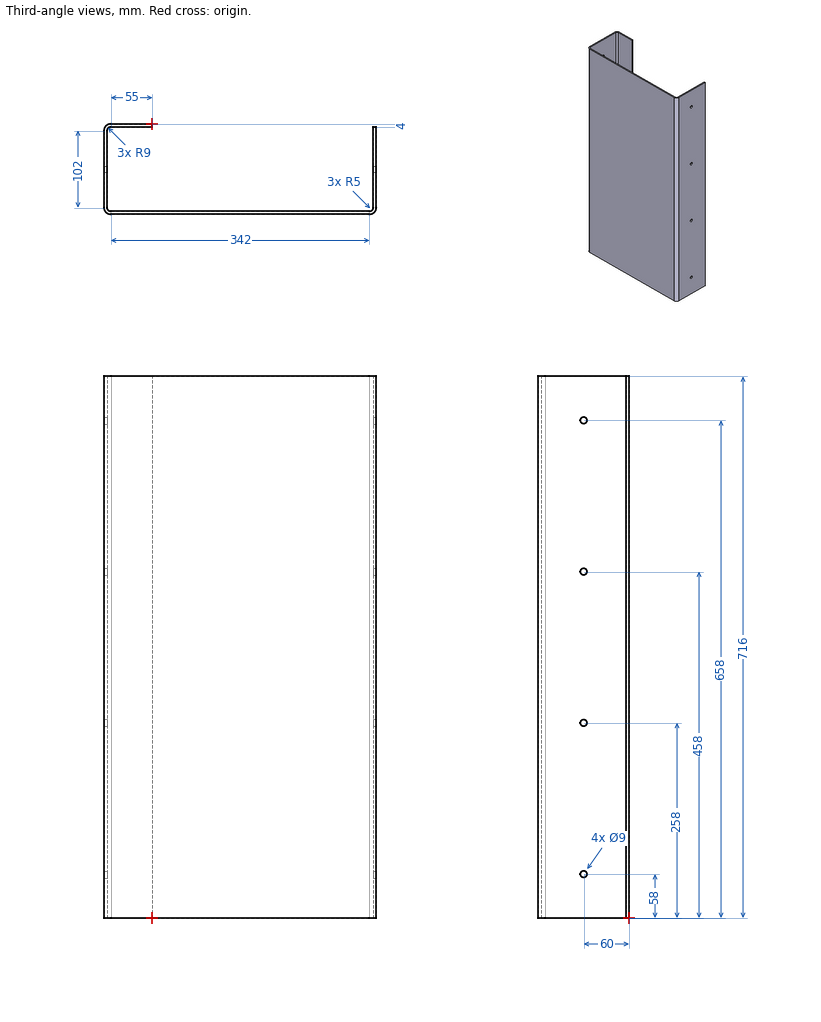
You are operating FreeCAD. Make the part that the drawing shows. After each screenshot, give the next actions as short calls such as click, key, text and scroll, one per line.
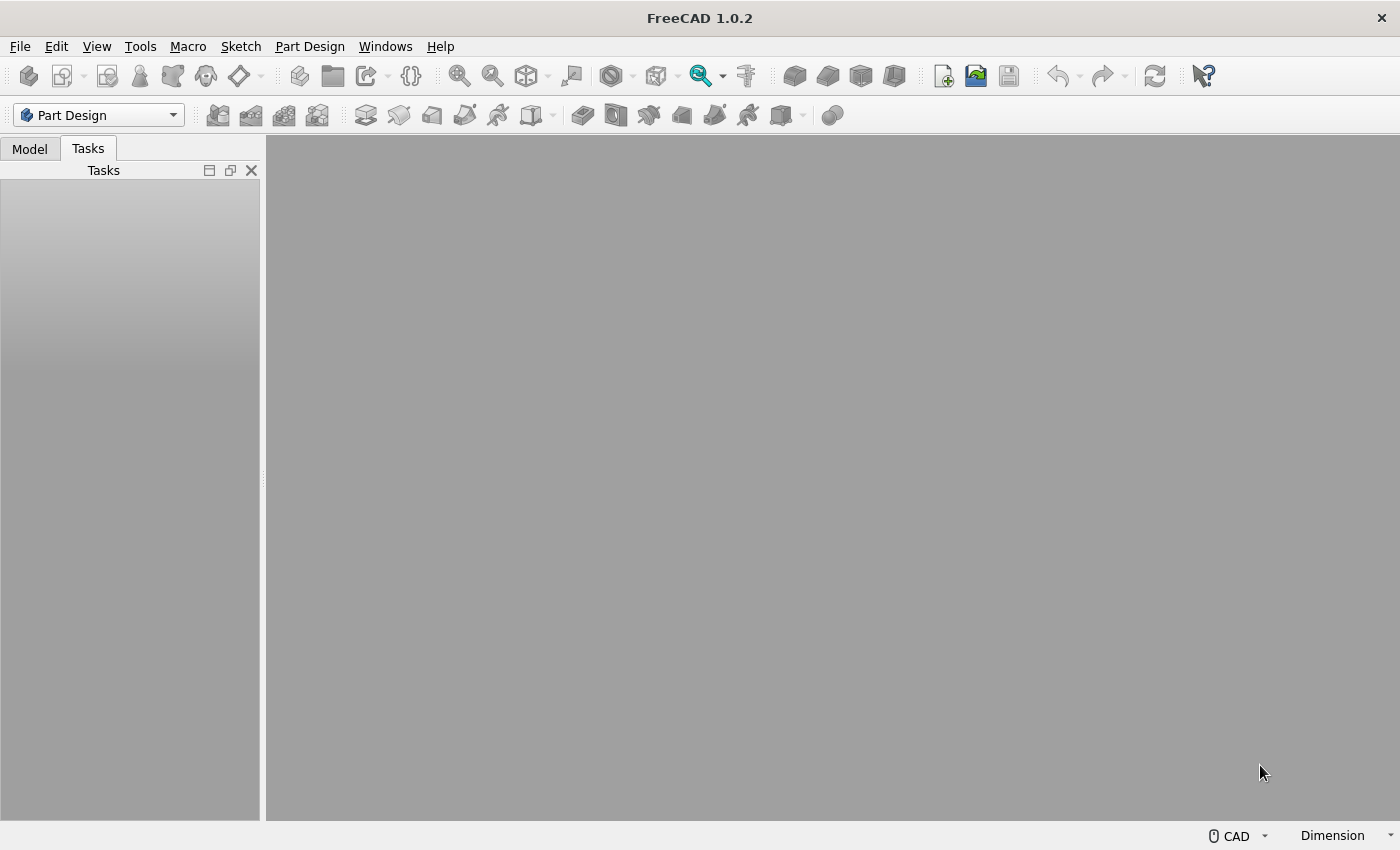
click(943, 76)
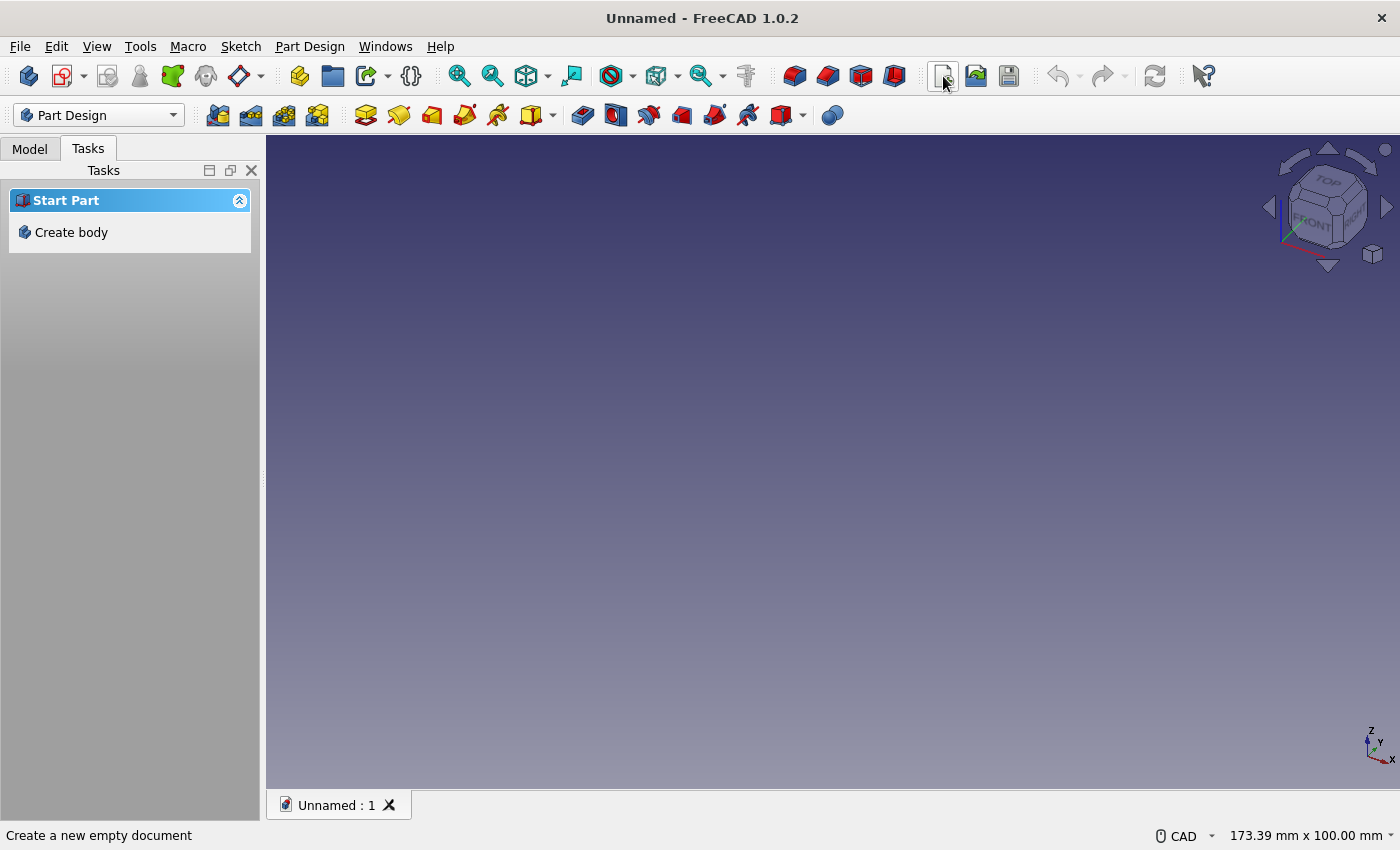
click(62, 76)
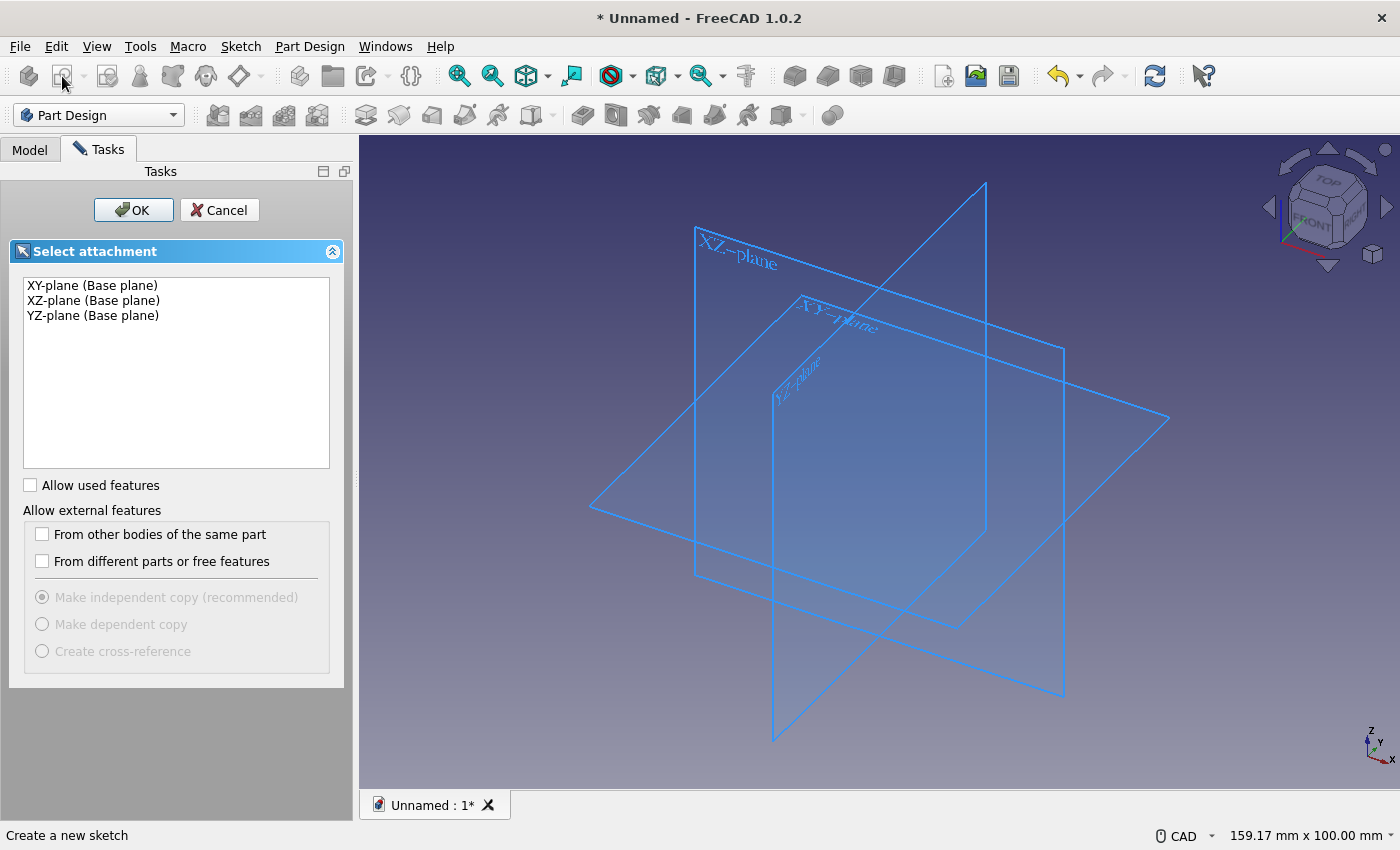
click(84, 286)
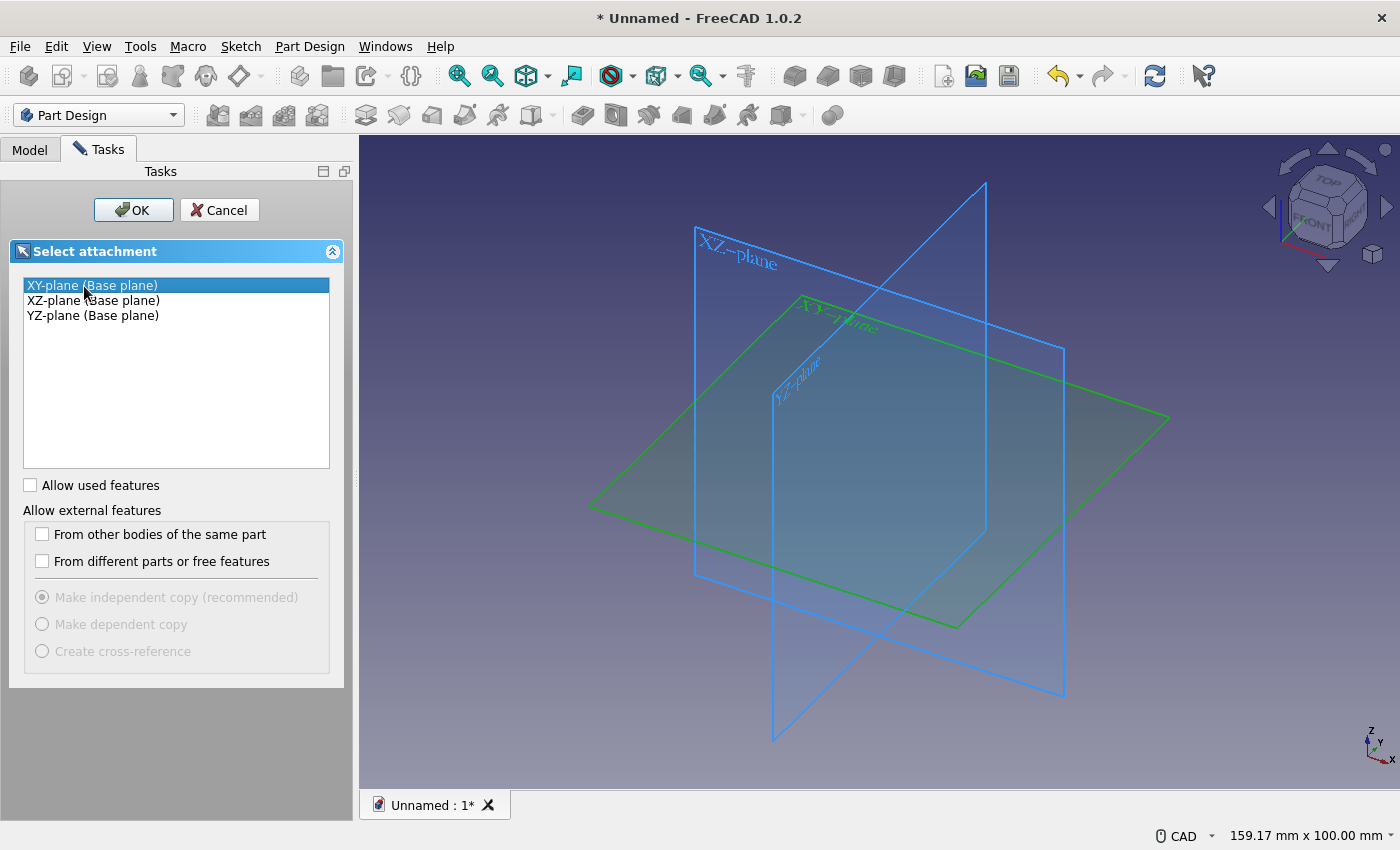
click(134, 210)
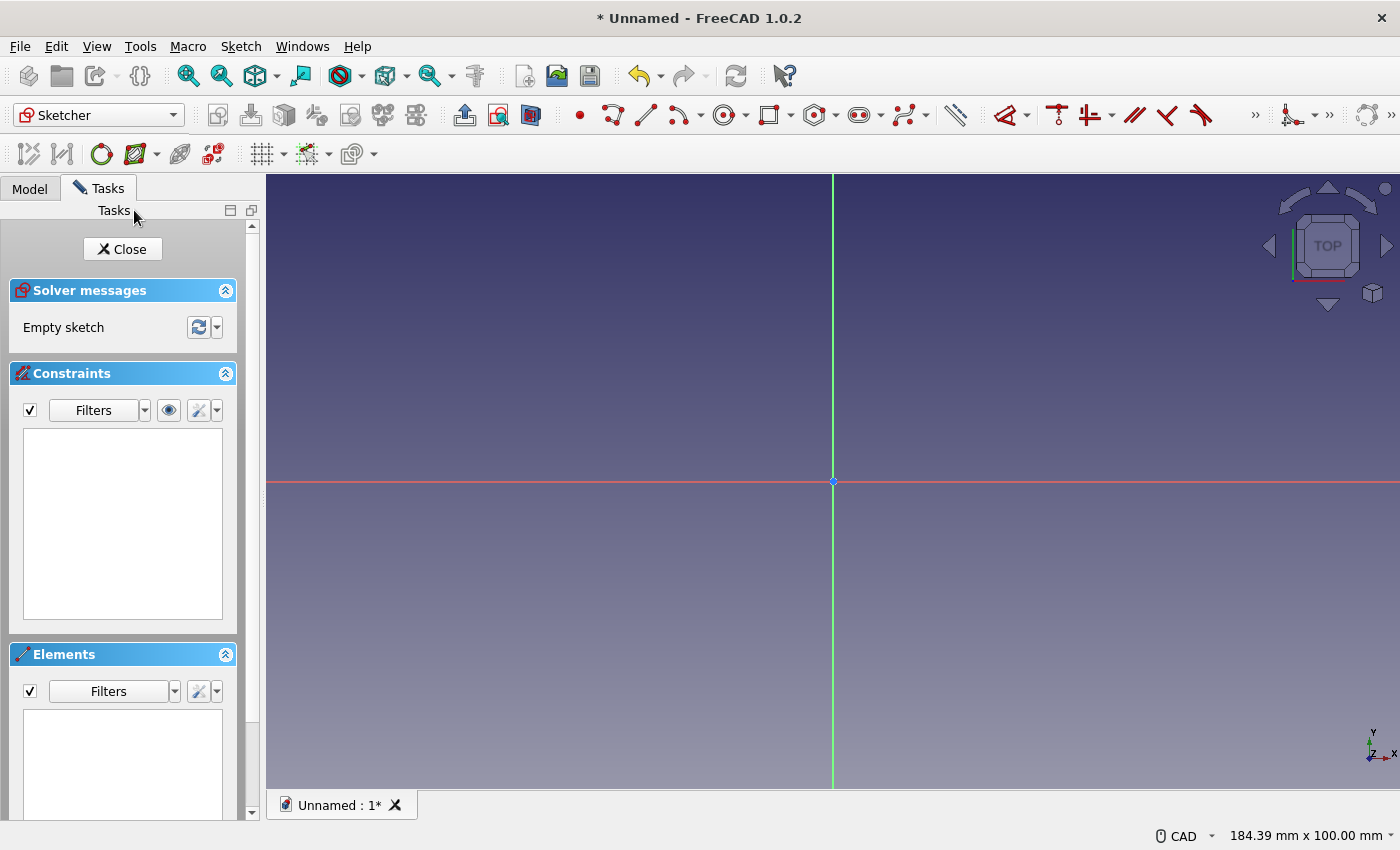
scroll(427, 322, down, 6)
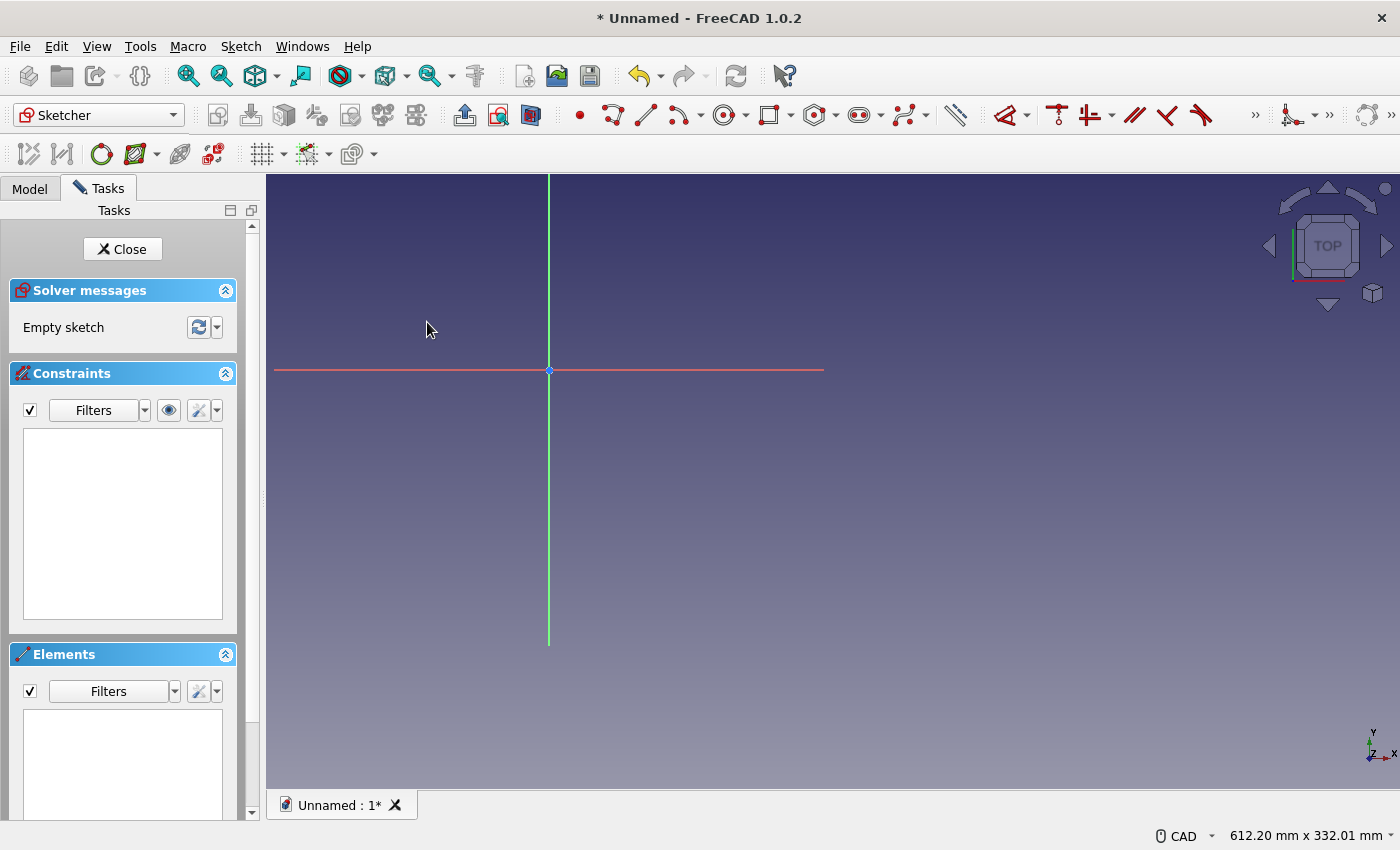
click(646, 116)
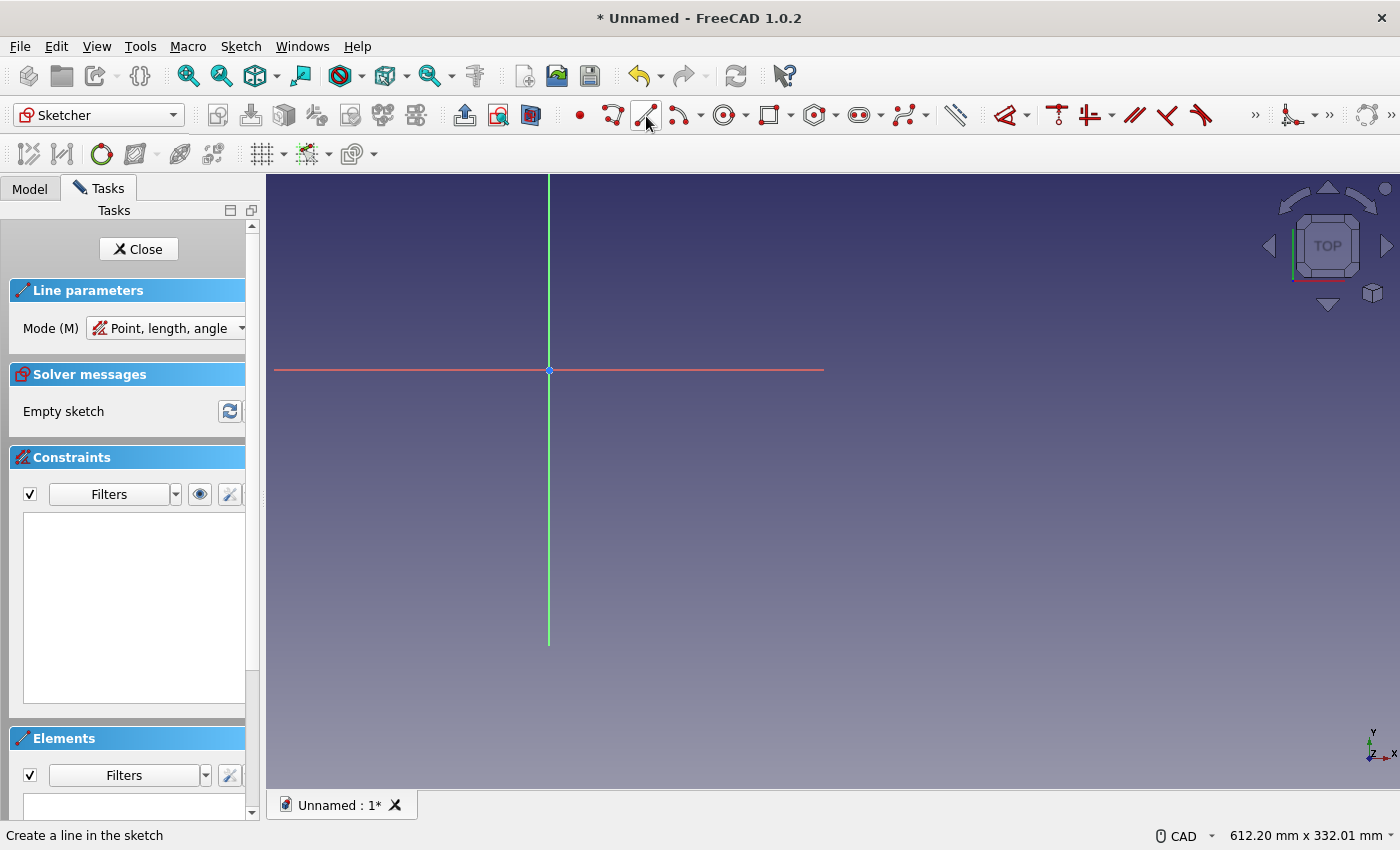
click(431, 387)
click(431, 576)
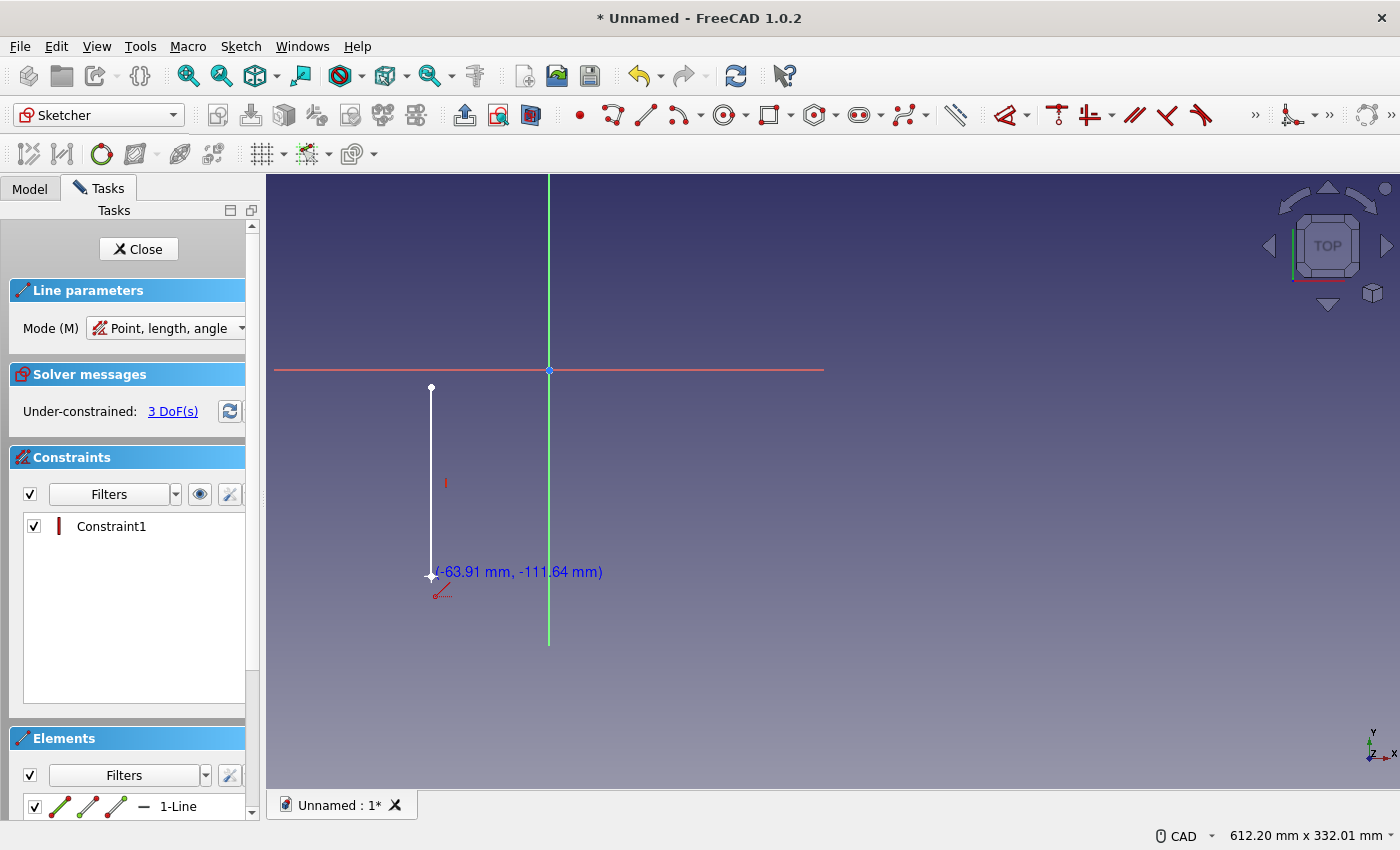
click(448, 592)
click(1081, 592)